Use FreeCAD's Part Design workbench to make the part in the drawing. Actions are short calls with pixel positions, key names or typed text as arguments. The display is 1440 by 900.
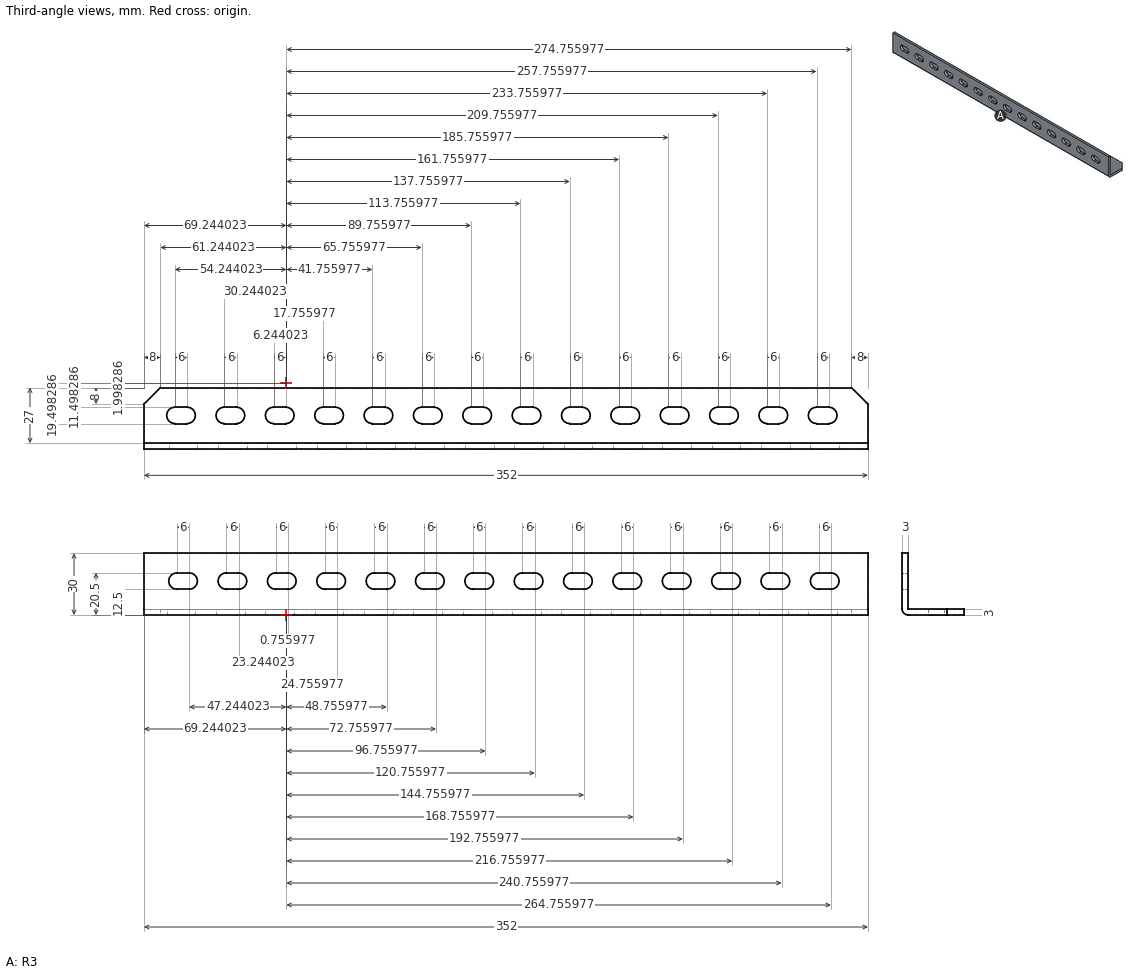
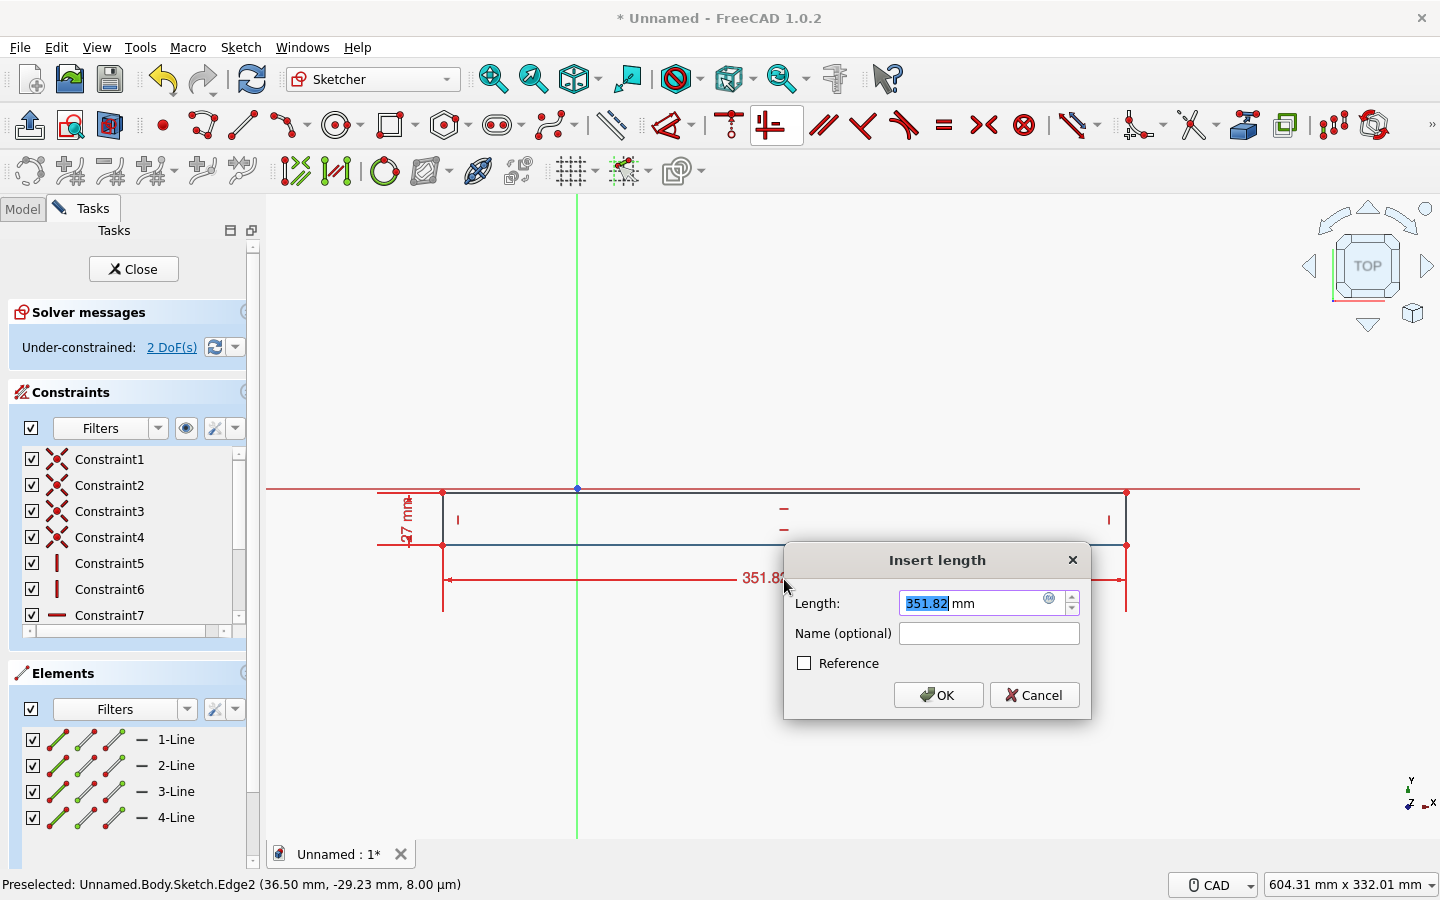
text(352)
key(Return)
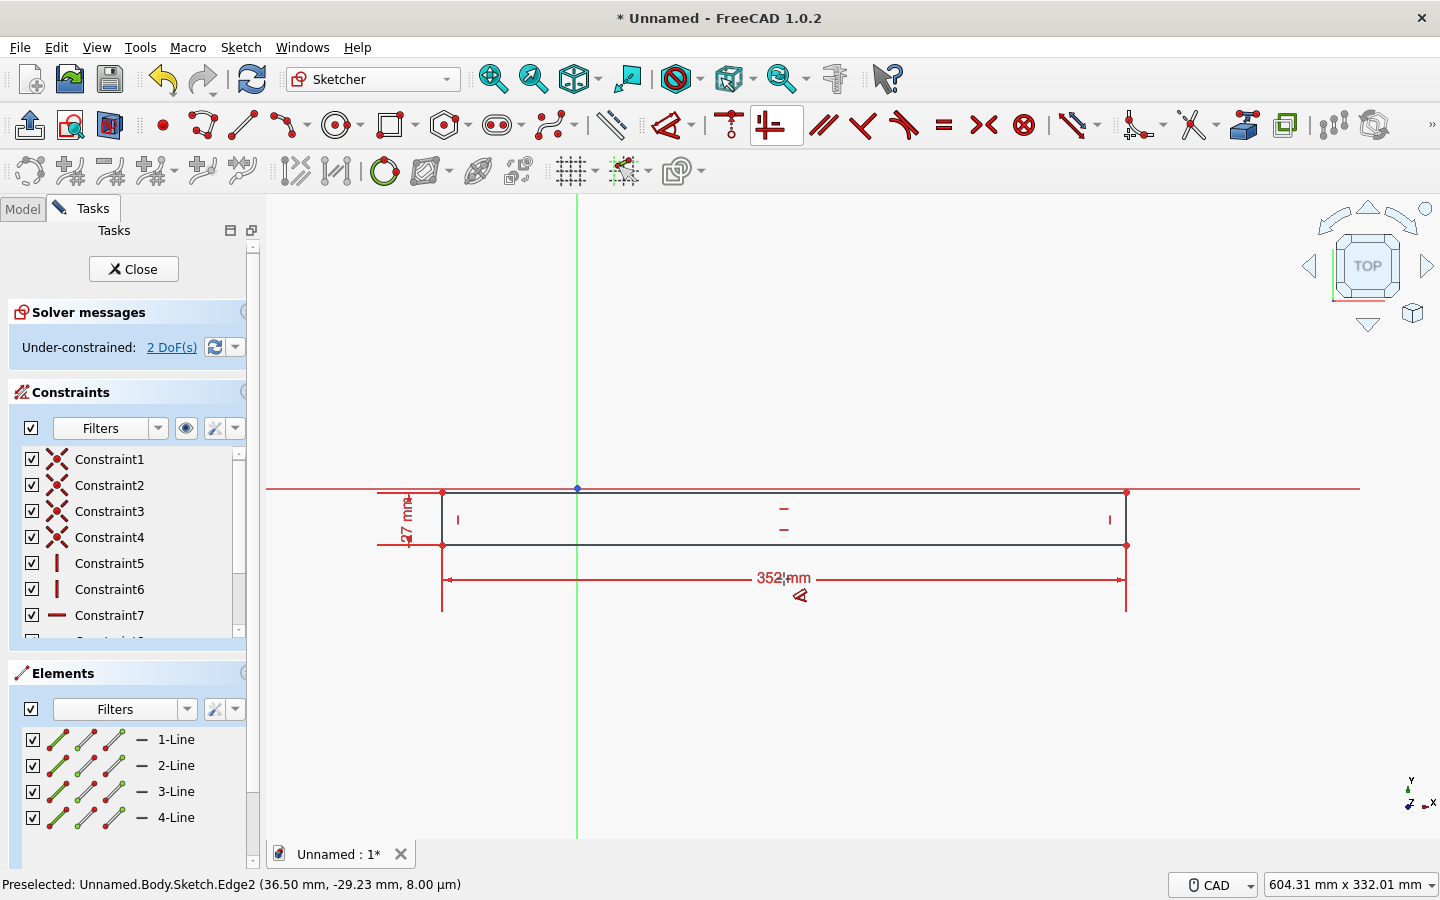
scroll(442, 493, up, 12)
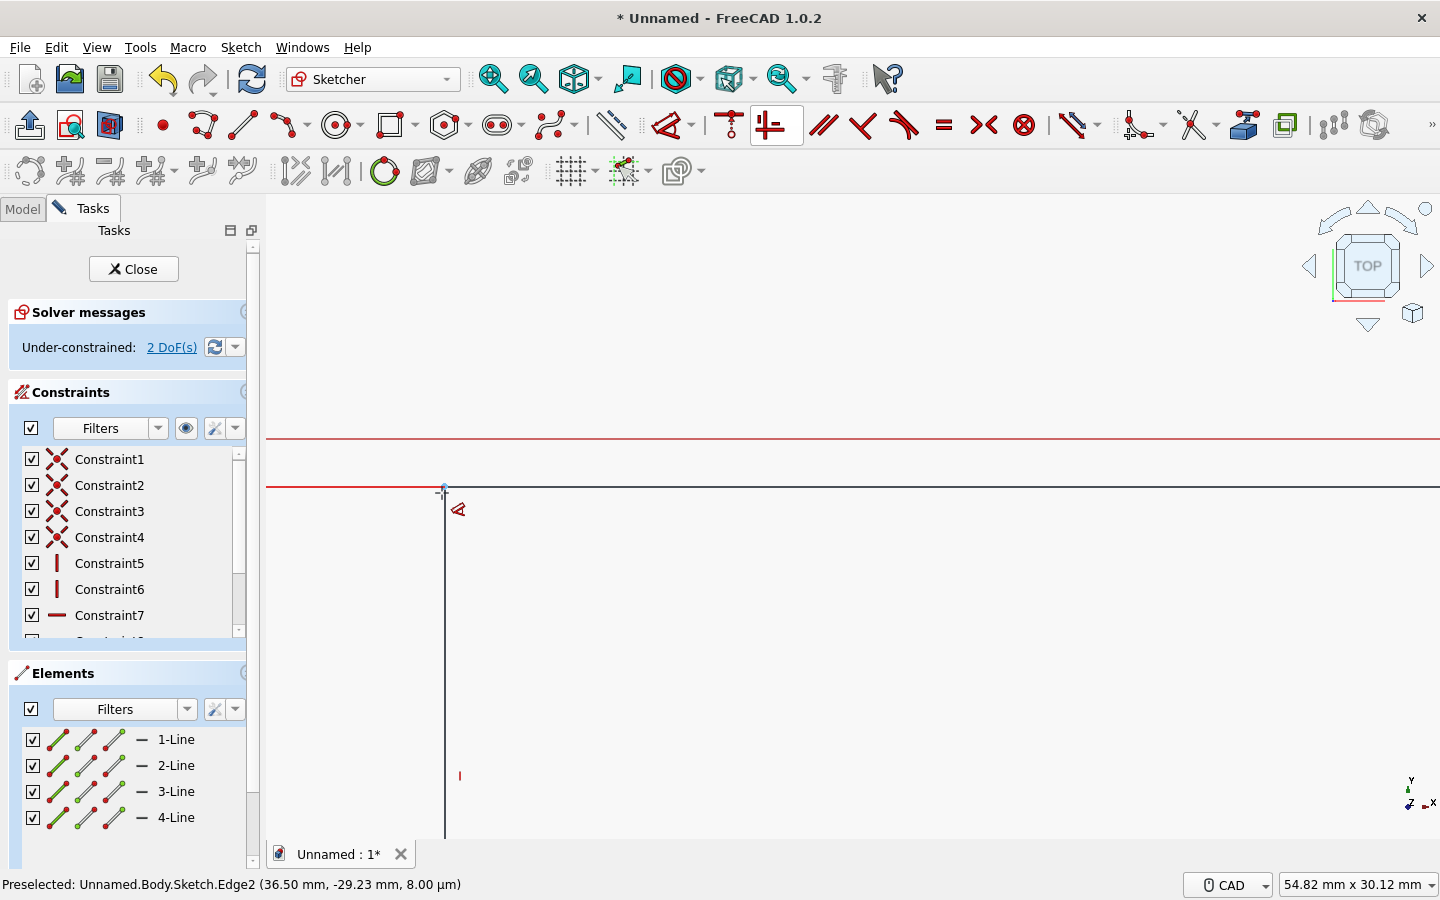
click(445, 487)
click(411, 463)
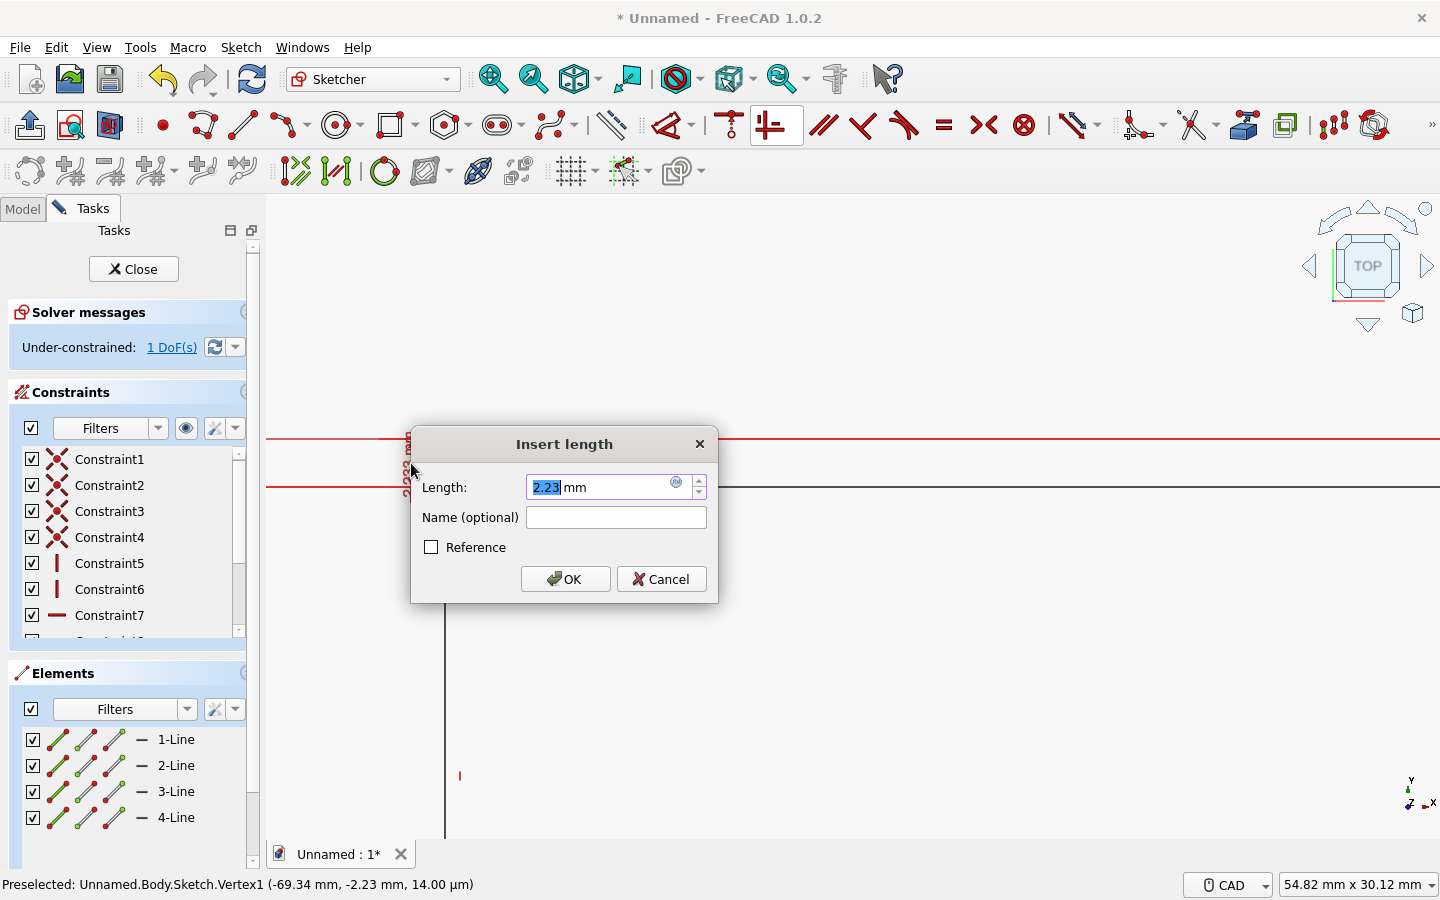
text(1.998286)
key(Return)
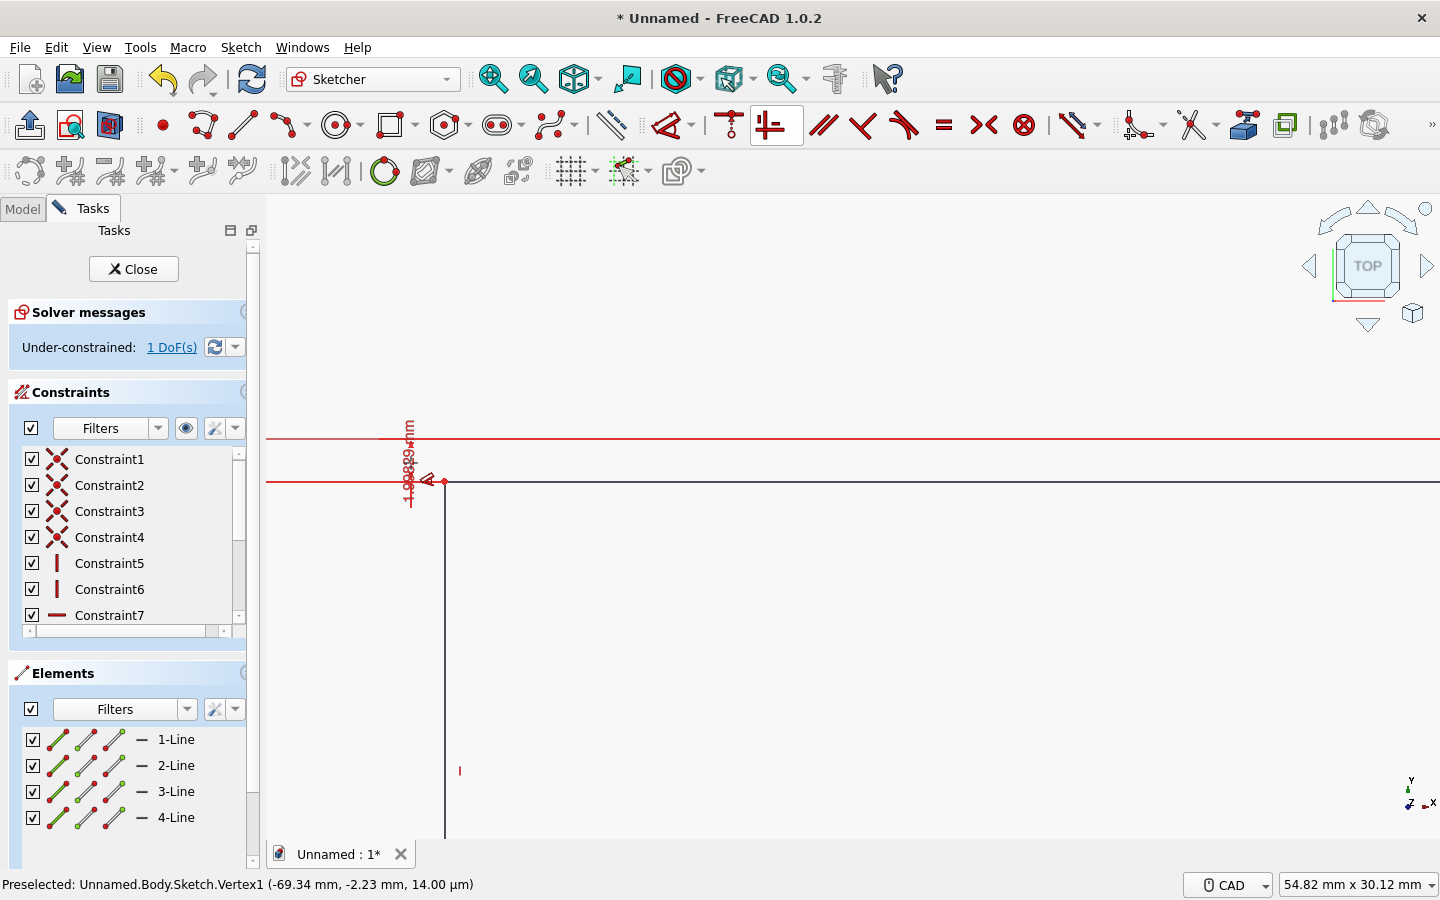
scroll(442, 493, down, 12)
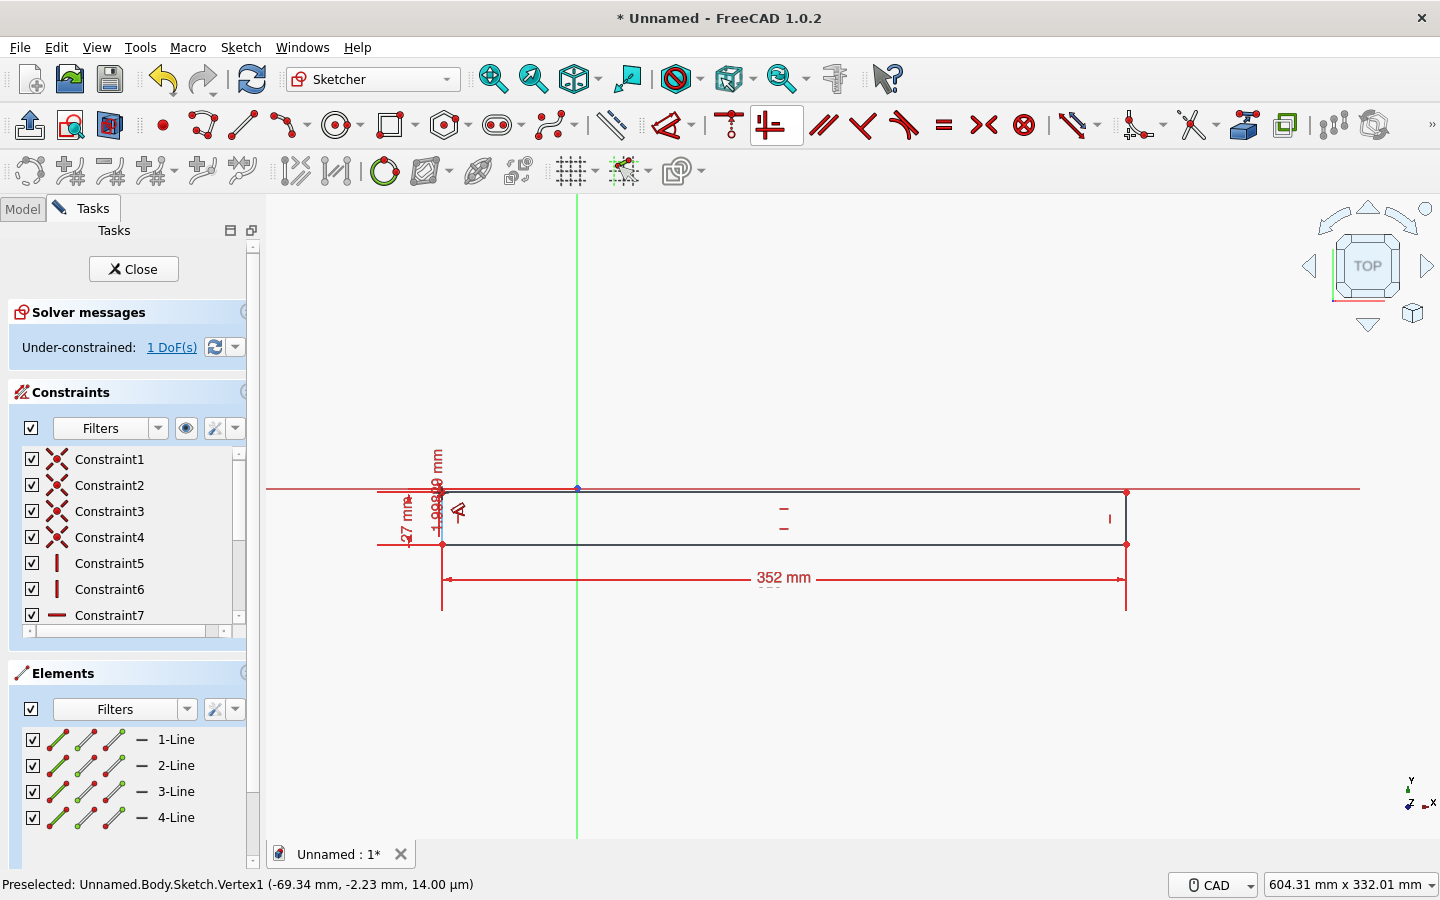
click(442, 492)
click(510, 455)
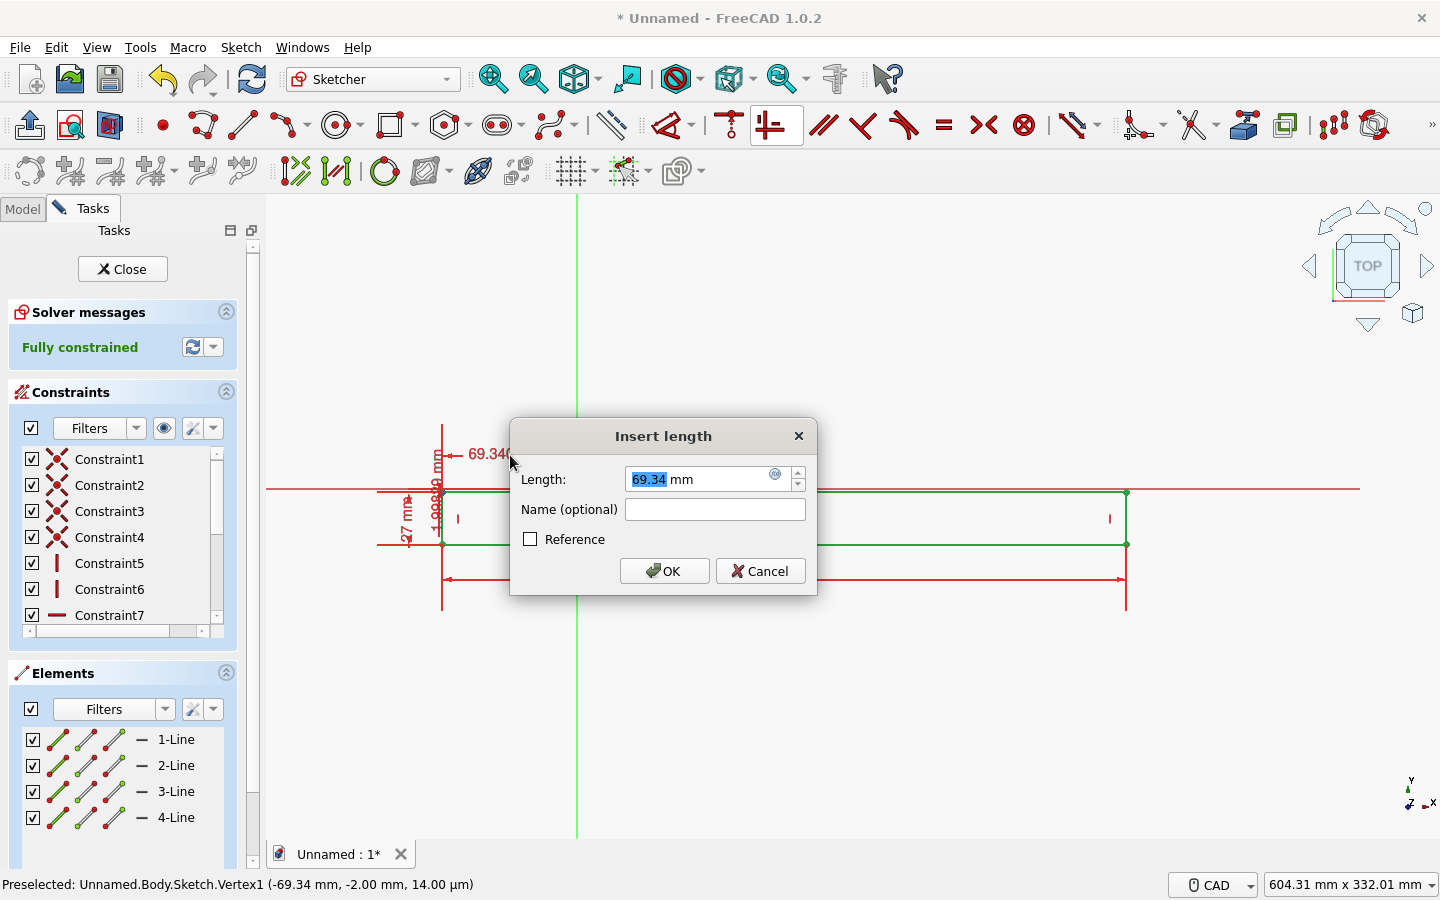
text(69.244023)
key(Return)
key(Escape)